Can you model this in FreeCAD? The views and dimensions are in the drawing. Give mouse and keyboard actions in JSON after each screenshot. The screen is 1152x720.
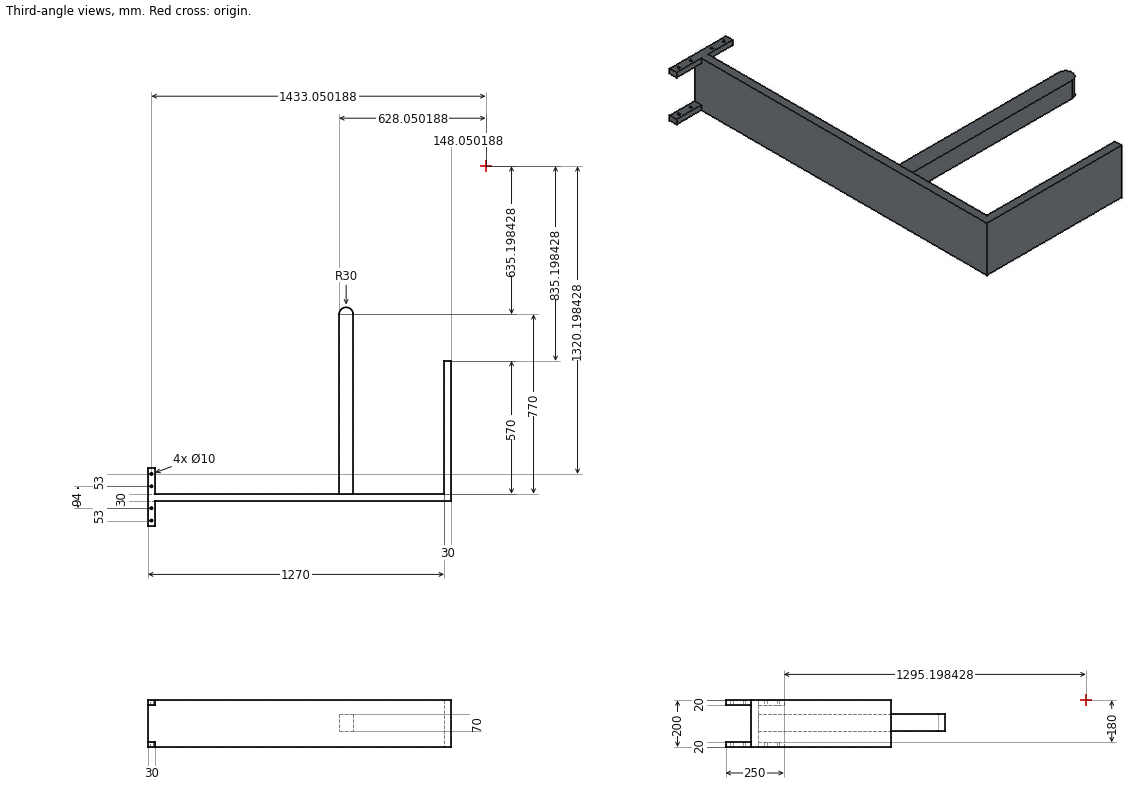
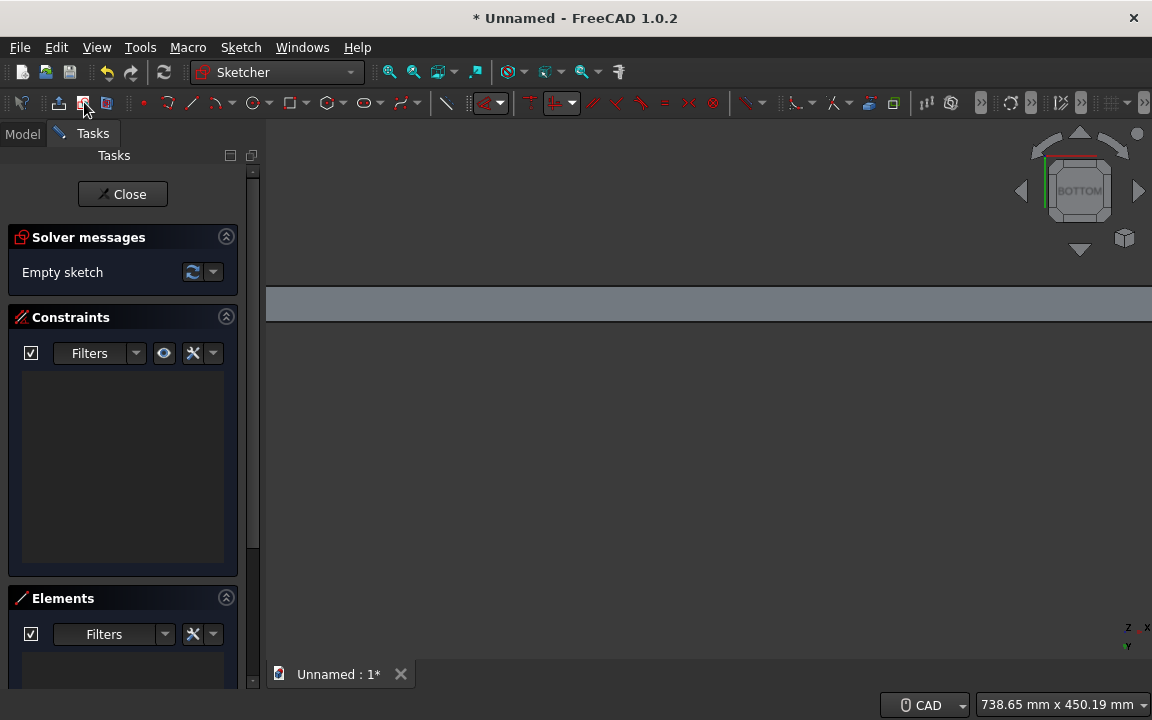
{"action": "scroll", "coordinate": [640, 389], "scroll_direction": "down", "scroll_amount": 5}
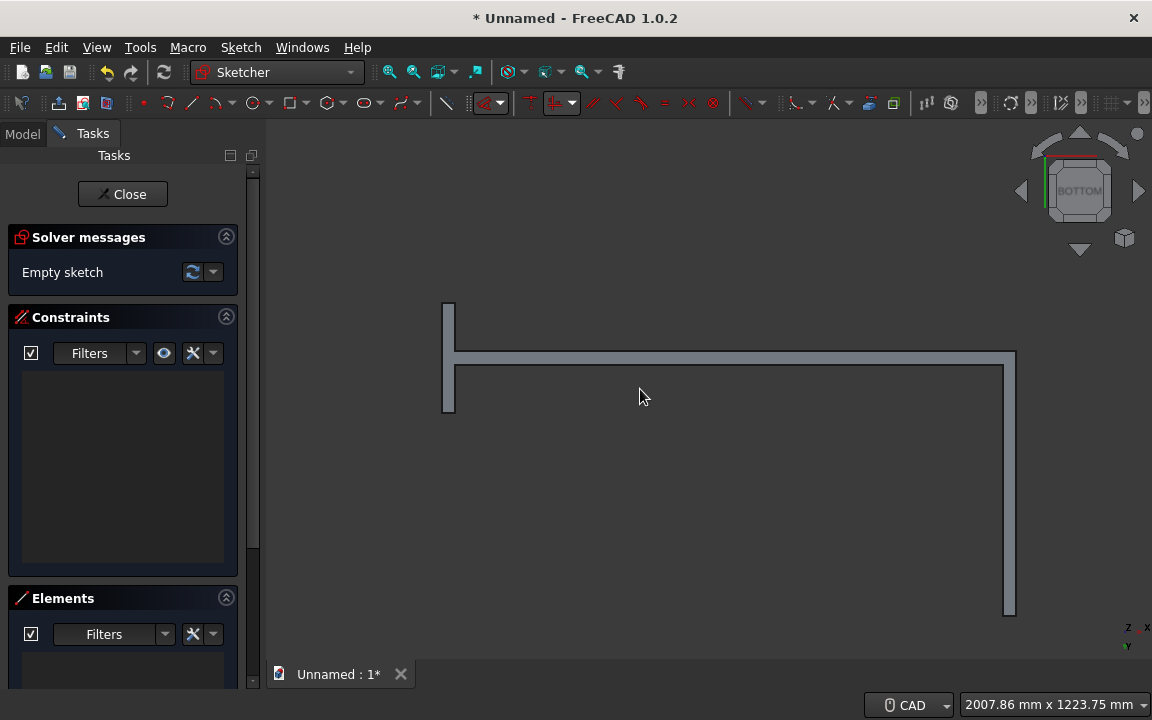
{"action": "scroll", "coordinate": [386, 348], "scroll_direction": "up", "scroll_amount": 7}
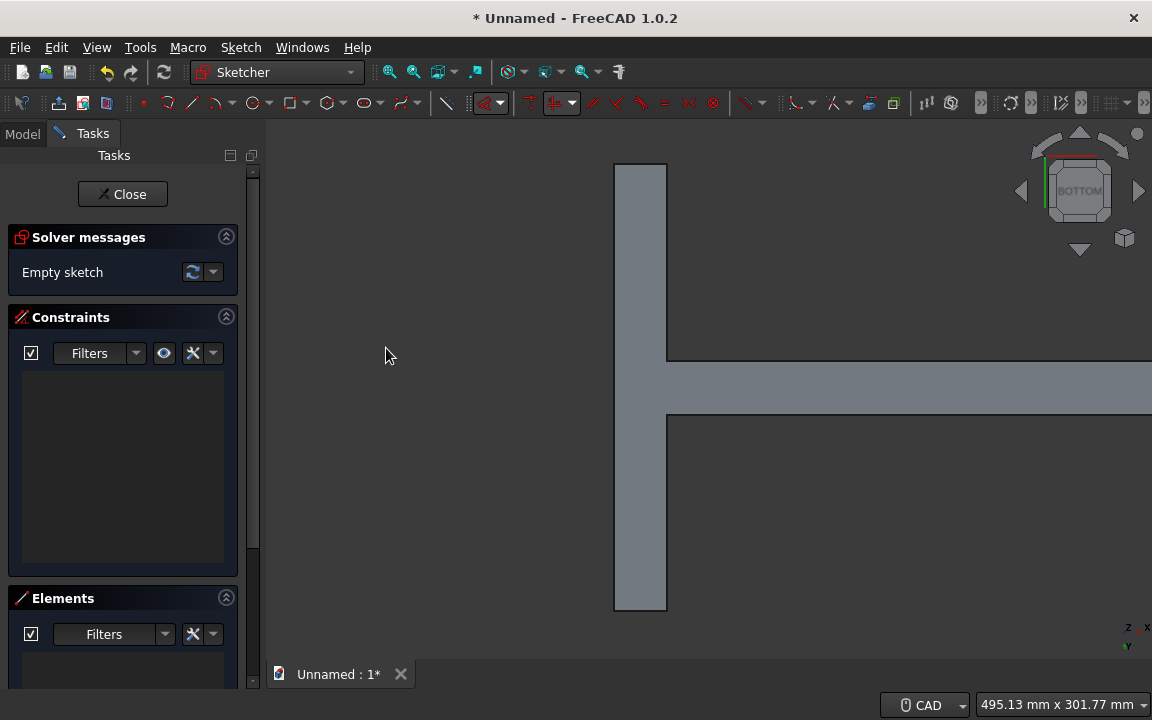
{"action": "left_click", "coordinate": [254, 104]}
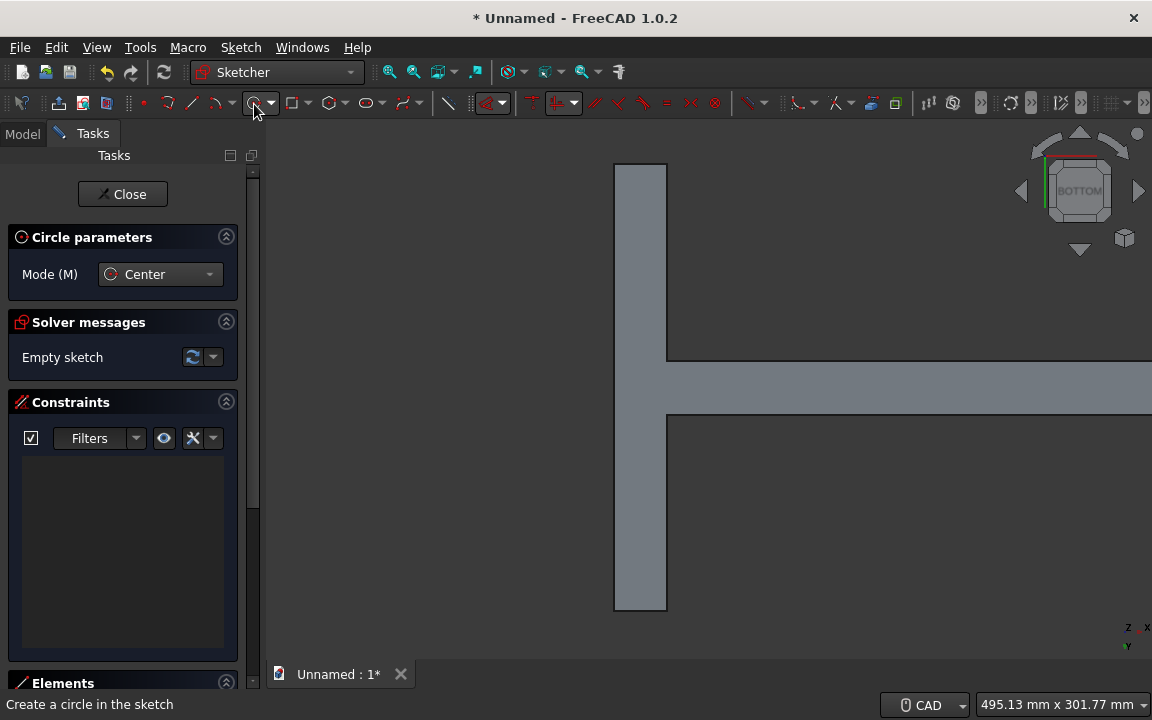
{"action": "scroll", "coordinate": [641, 567], "scroll_direction": "up", "scroll_amount": 5}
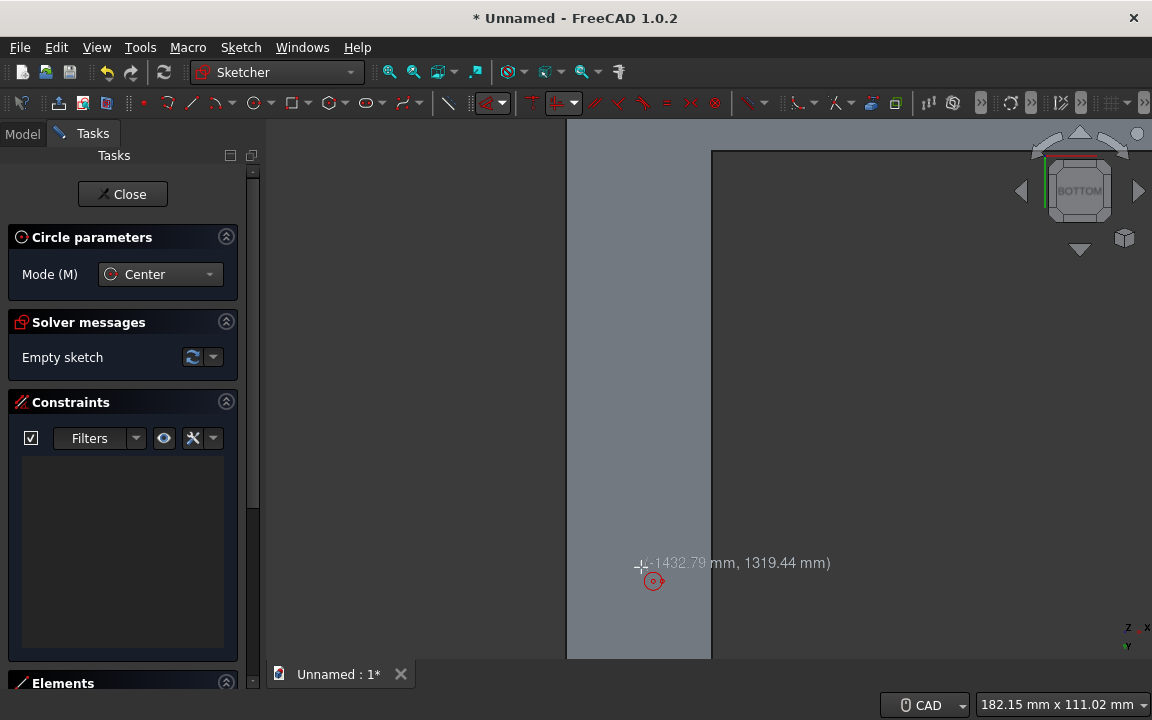
{"action": "left_click", "coordinate": [639, 565]}
{"action": "mouse_move", "coordinate": [656, 547]}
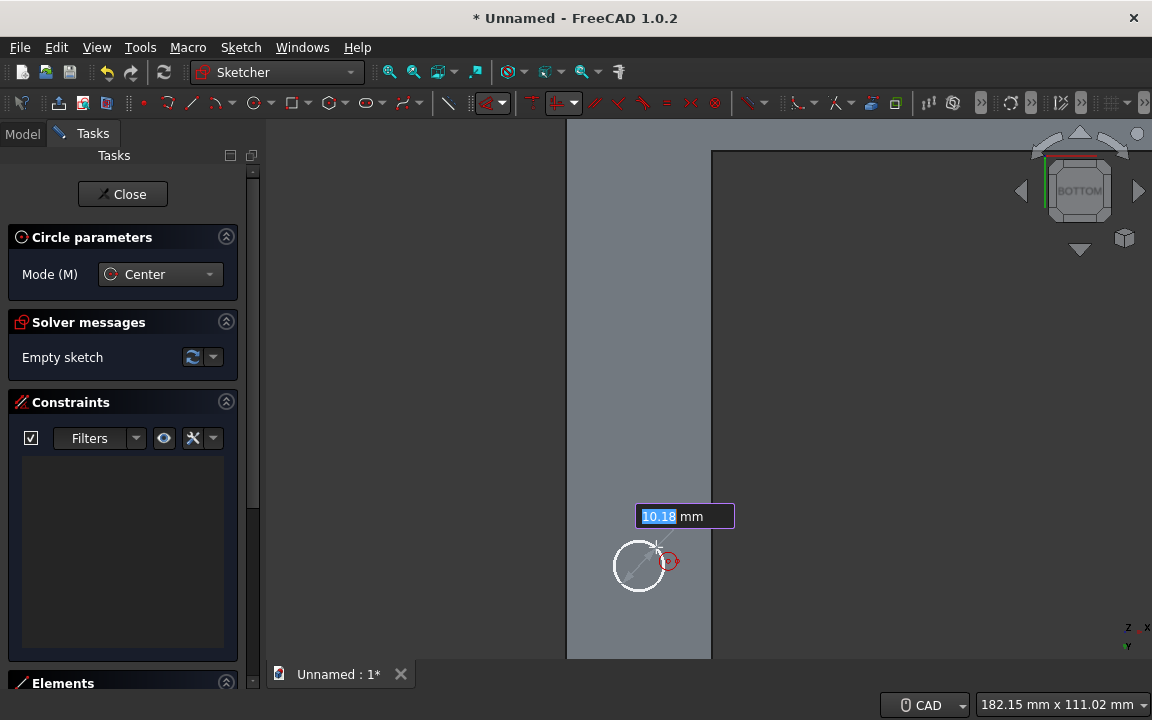
{"action": "type", "text": "10"}
{"action": "key", "text": "Return"}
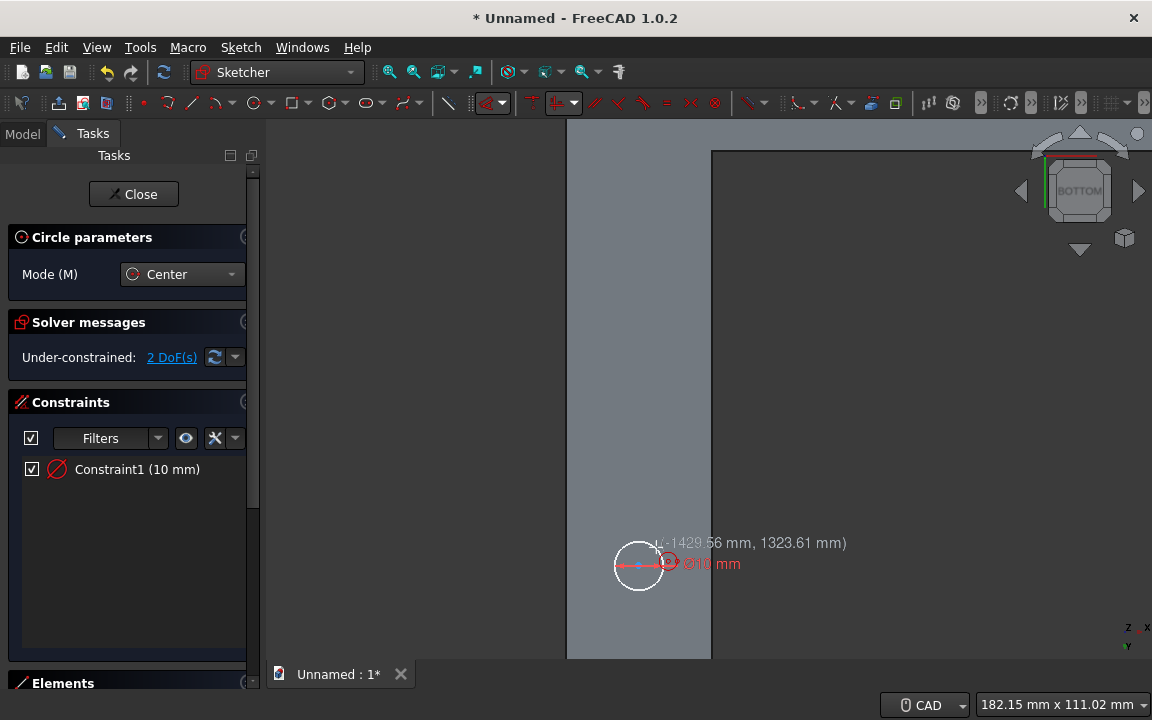
{"action": "left_click", "coordinate": [639, 307]}
{"action": "mouse_move", "coordinate": [656, 290]}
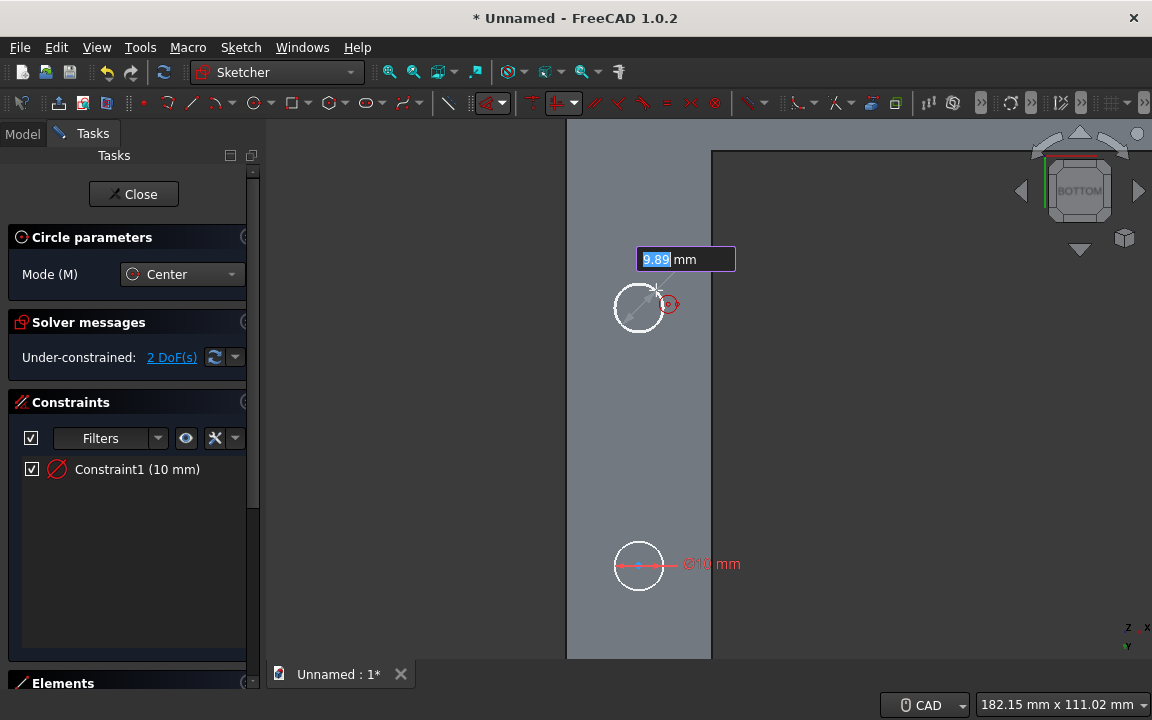
{"action": "type", "text": "10"}
{"action": "key", "text": "Return"}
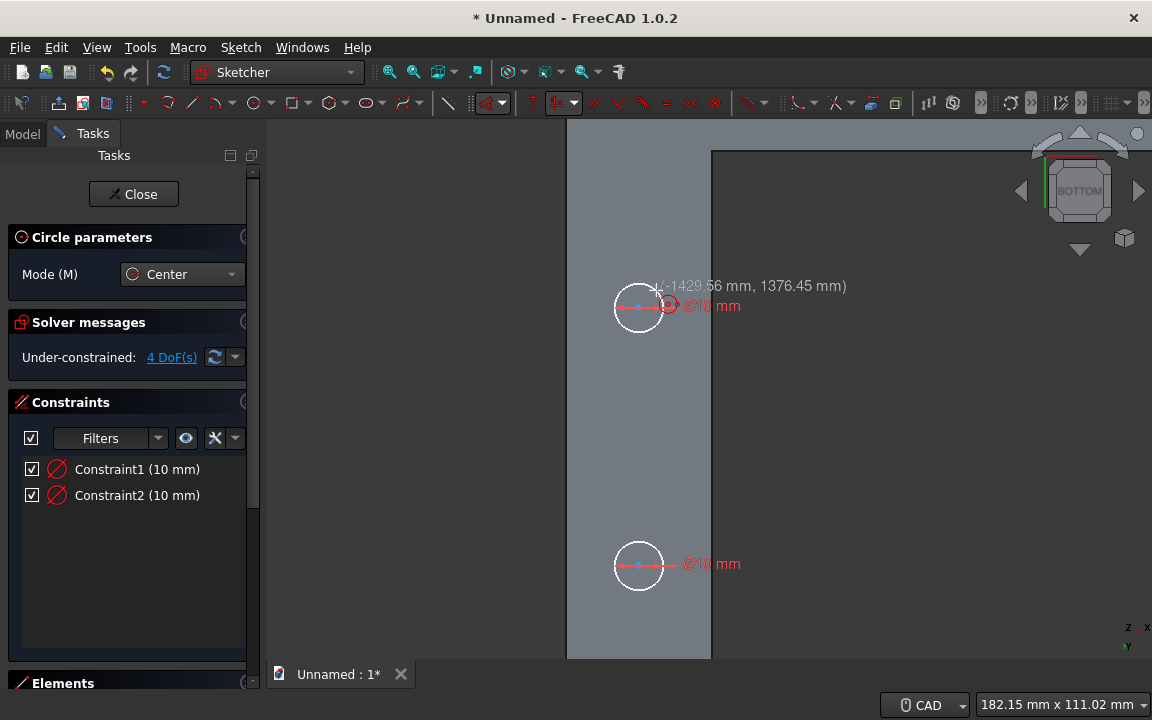
{"action": "scroll", "coordinate": [641, 570], "scroll_direction": "down", "scroll_amount": 5}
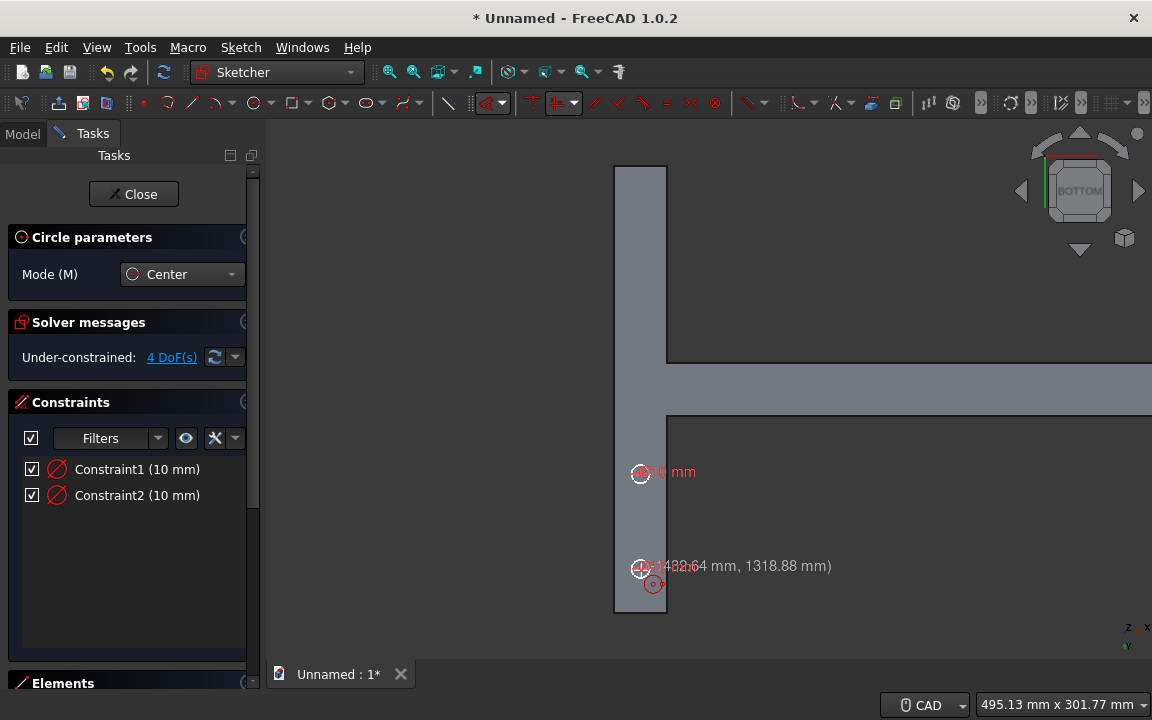
{"action": "scroll", "coordinate": [641, 211], "scroll_direction": "up", "scroll_amount": 5}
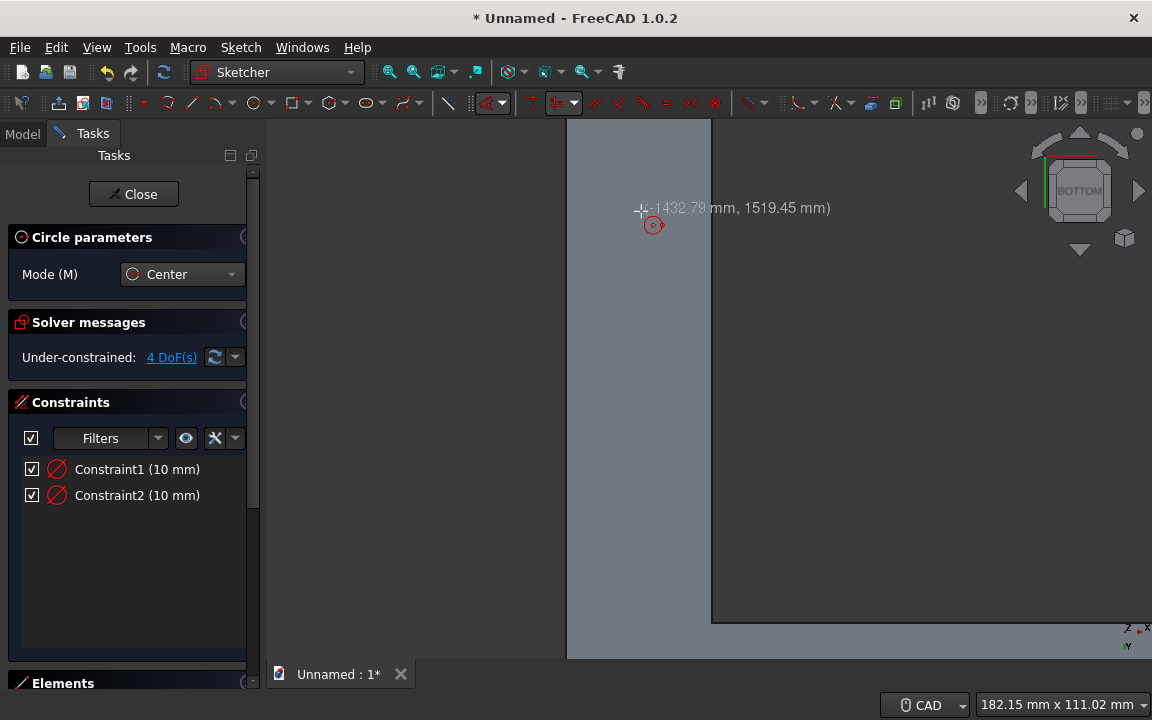
{"action": "left_click", "coordinate": [639, 210]}
{"action": "mouse_move", "coordinate": [656, 193]}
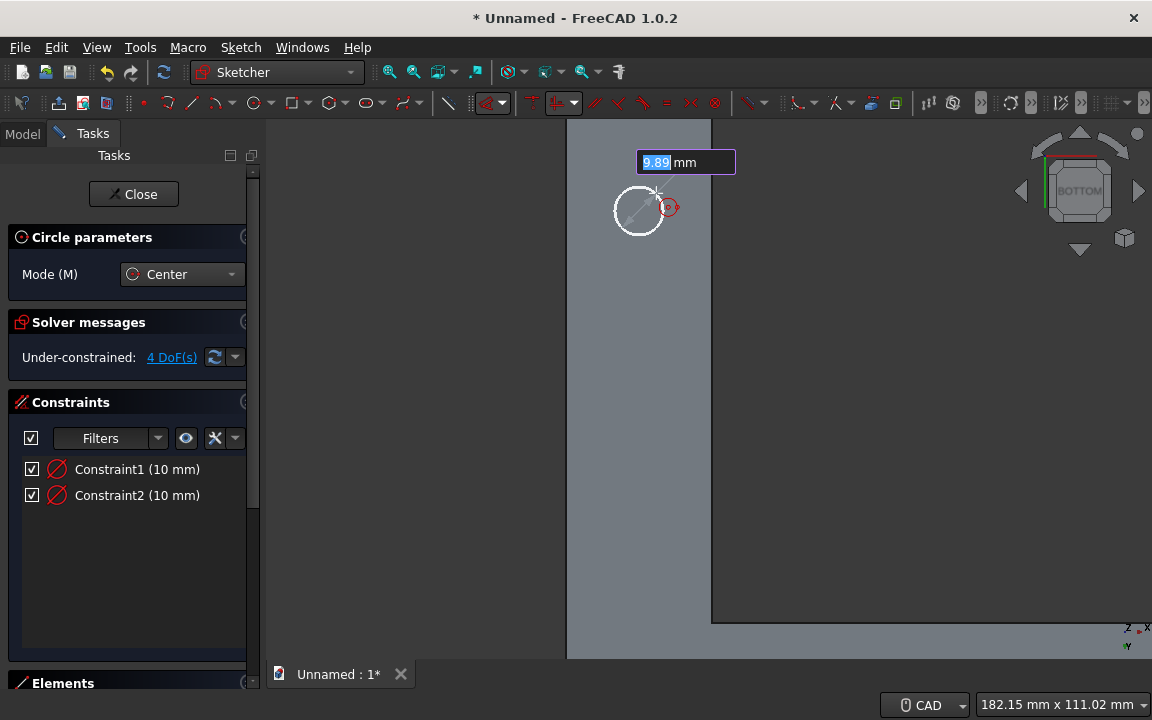
{"action": "type", "text": "10"}
{"action": "key", "text": "Return"}